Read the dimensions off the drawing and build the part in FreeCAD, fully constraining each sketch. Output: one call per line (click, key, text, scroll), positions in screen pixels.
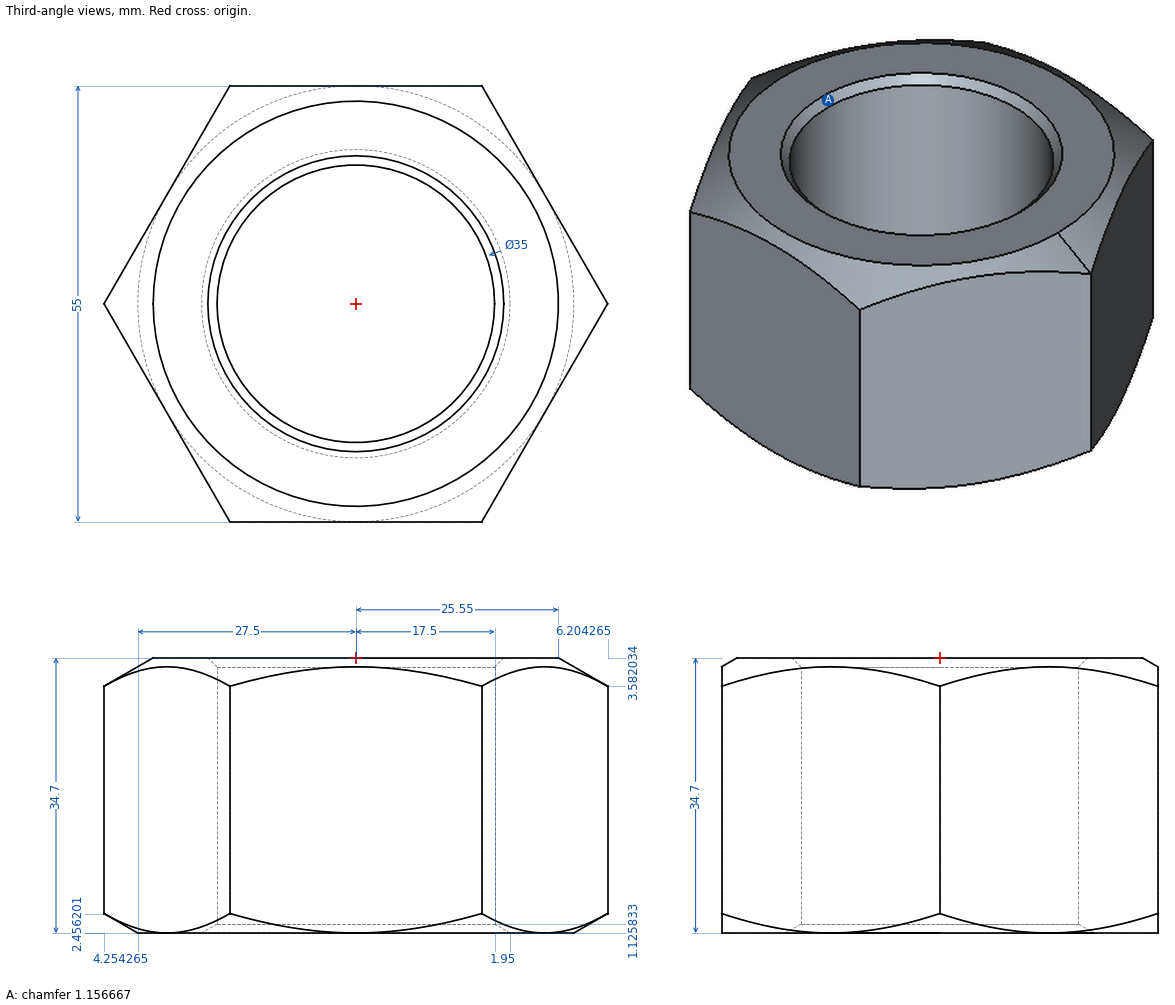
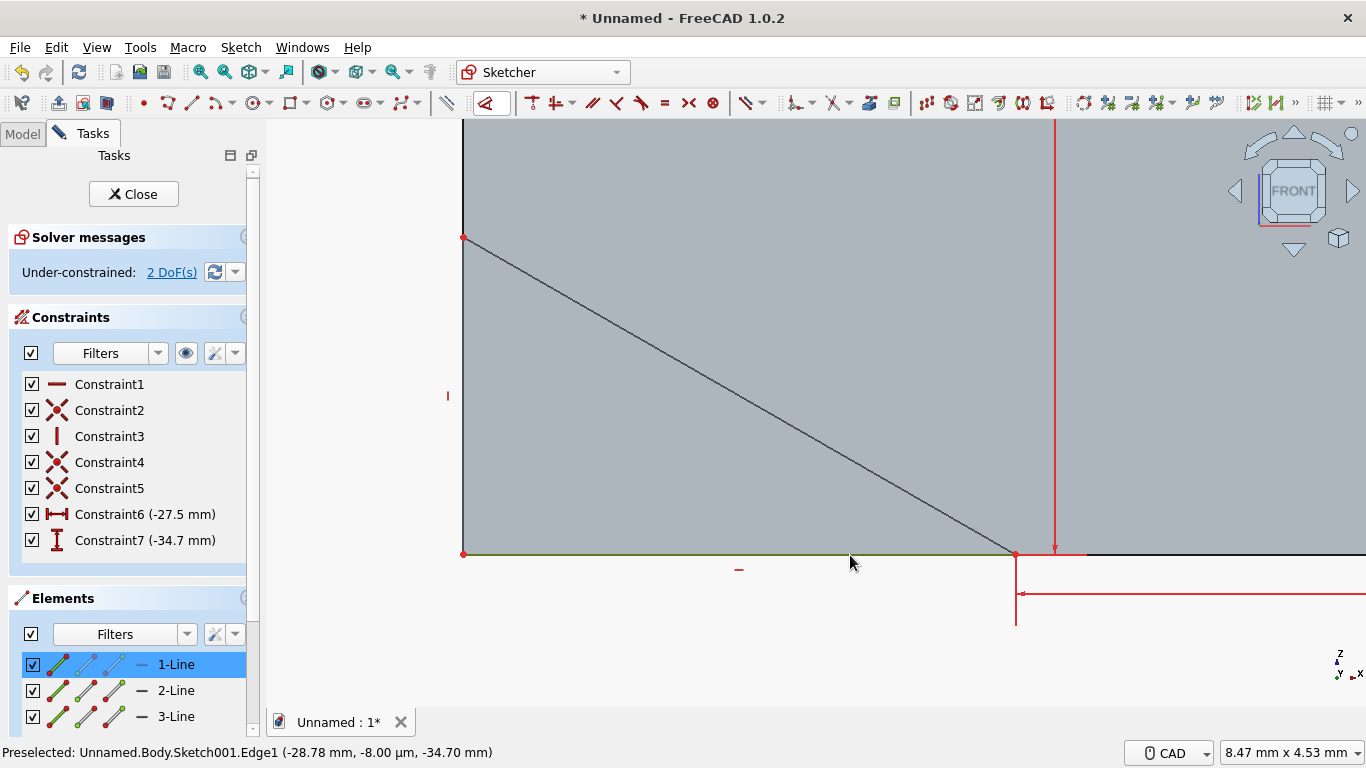
key(l)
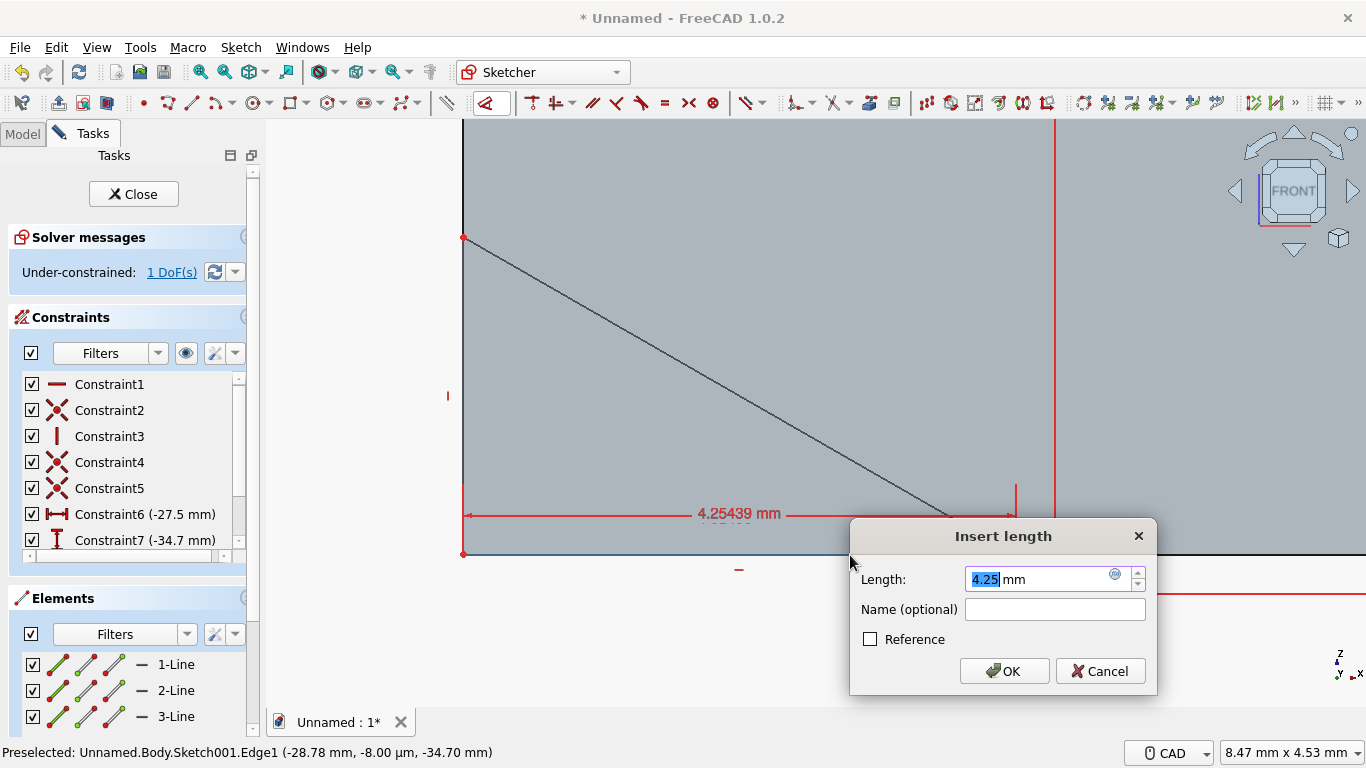
text(4.254265)
key(Return)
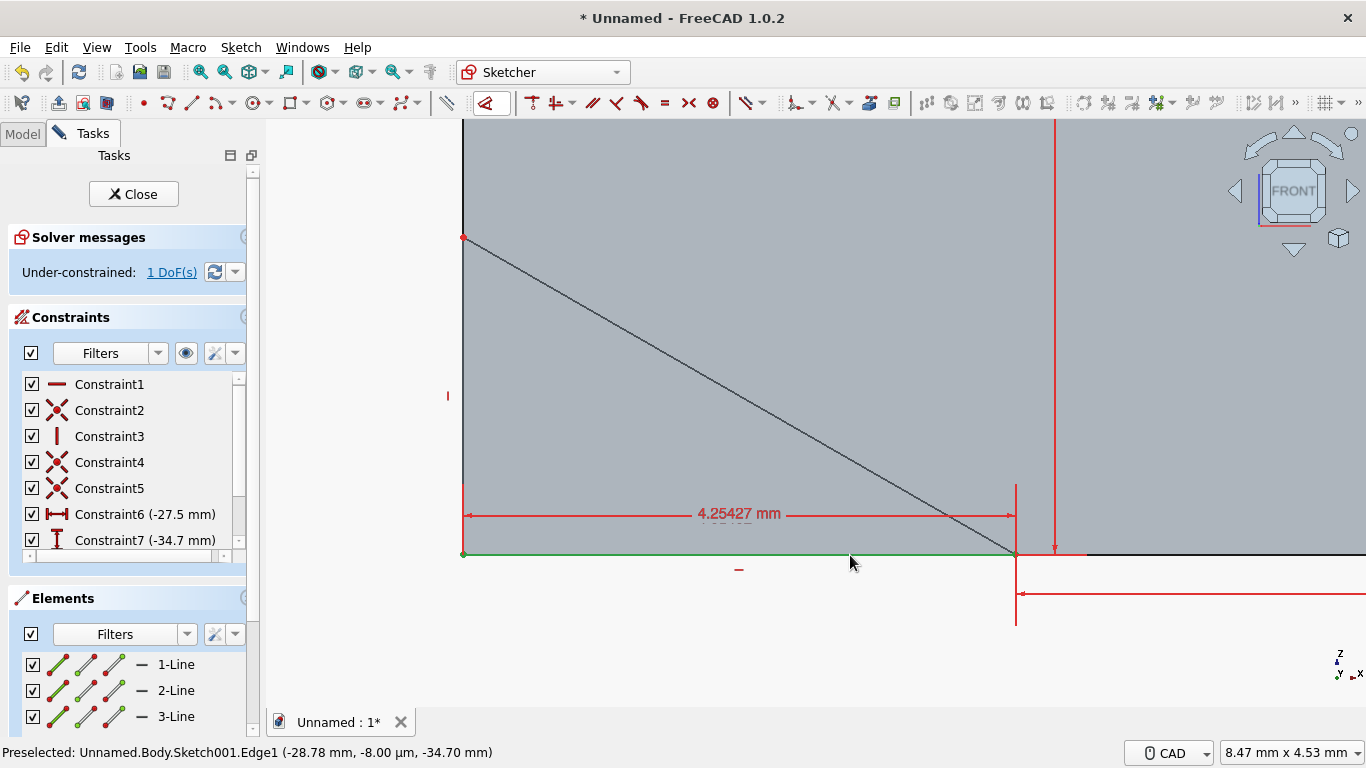
click(463, 459)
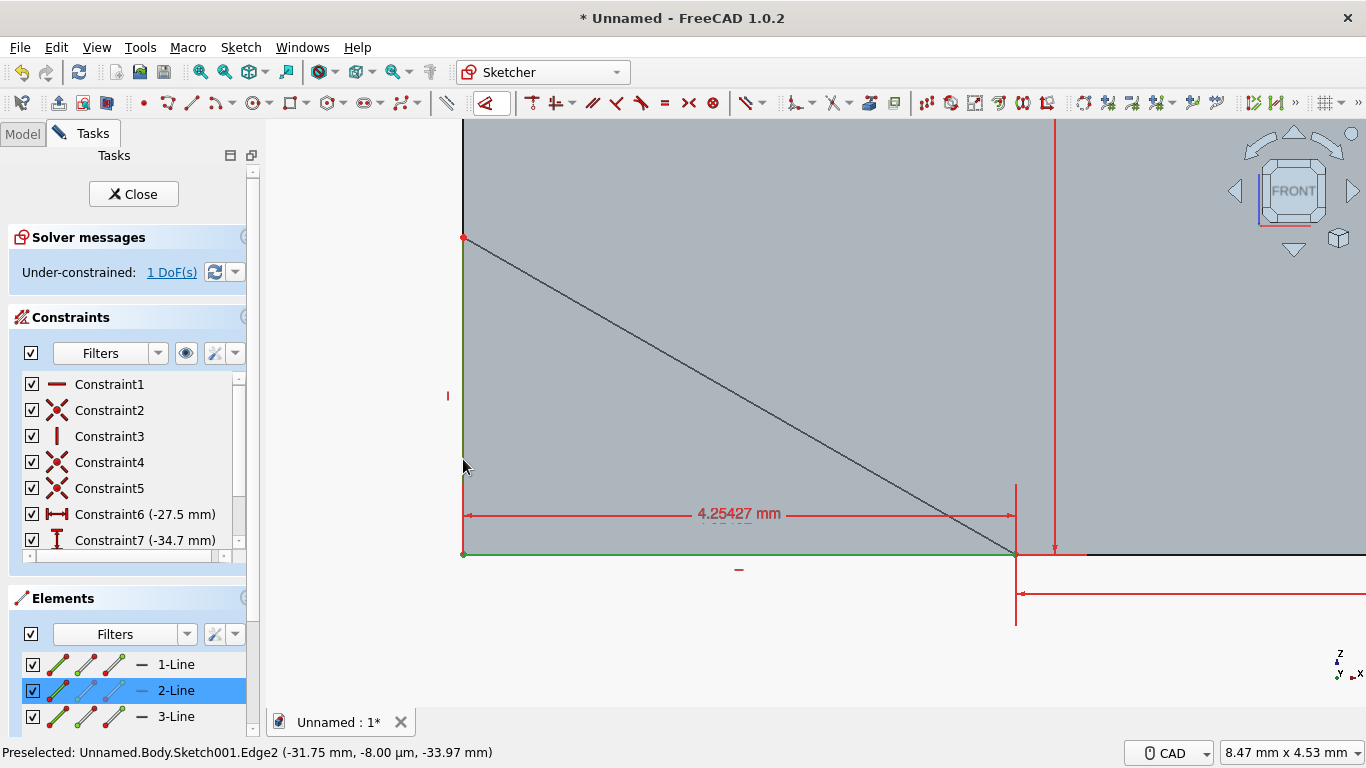
key(i)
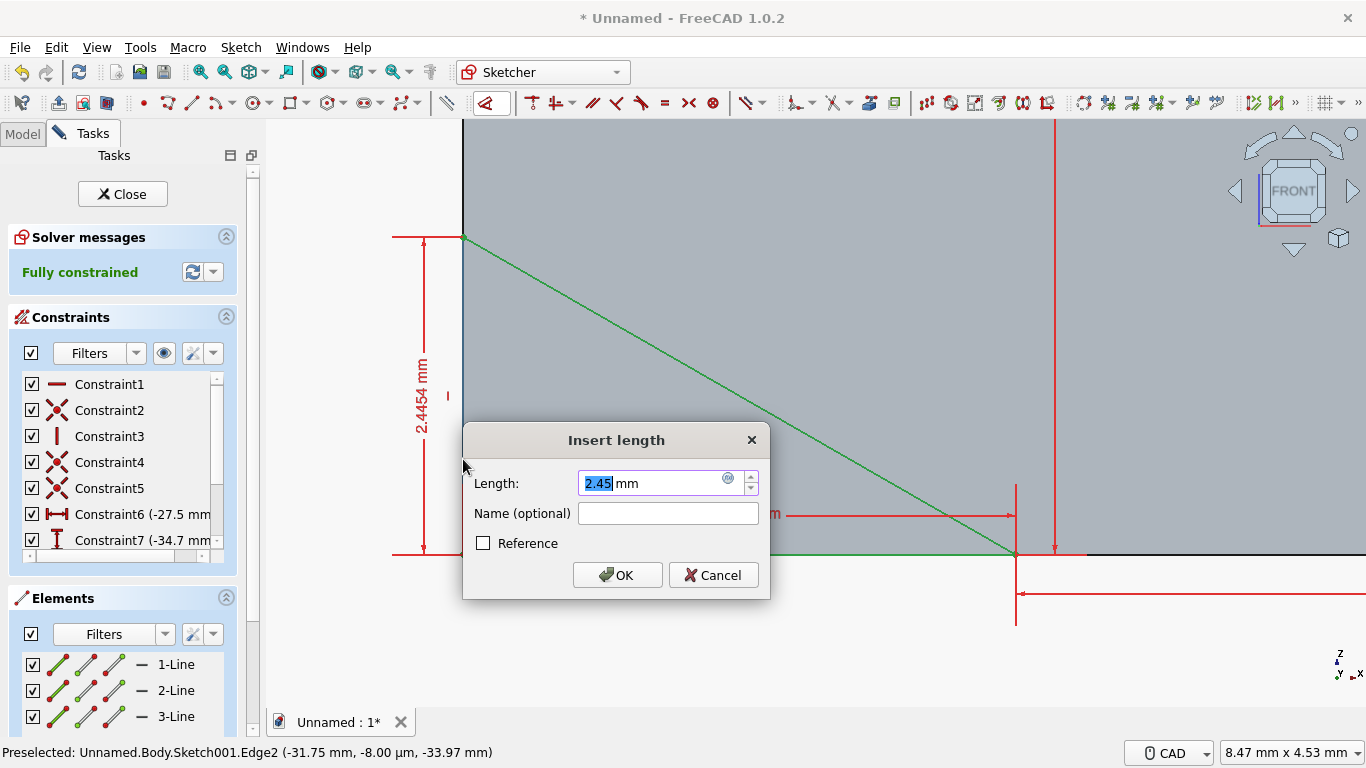
text(2.456201)
key(Return)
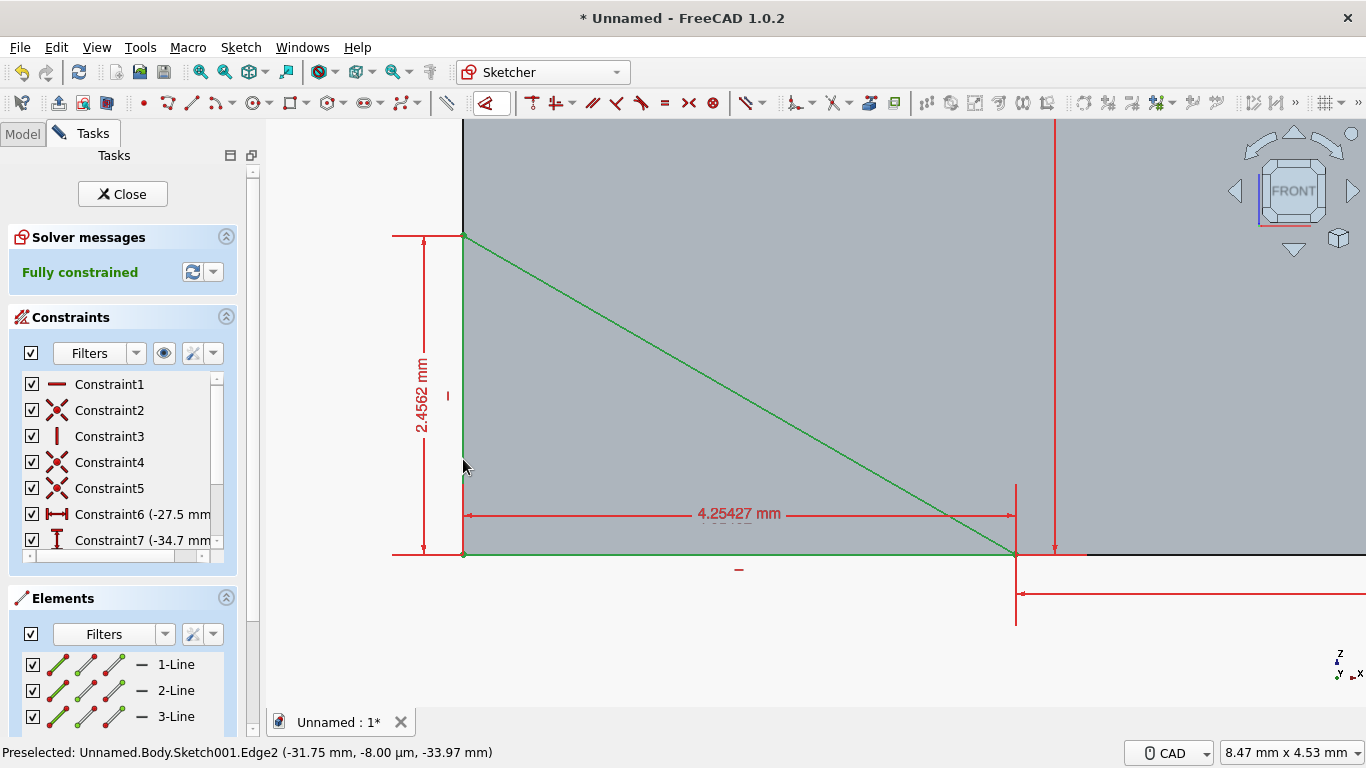
click(123, 194)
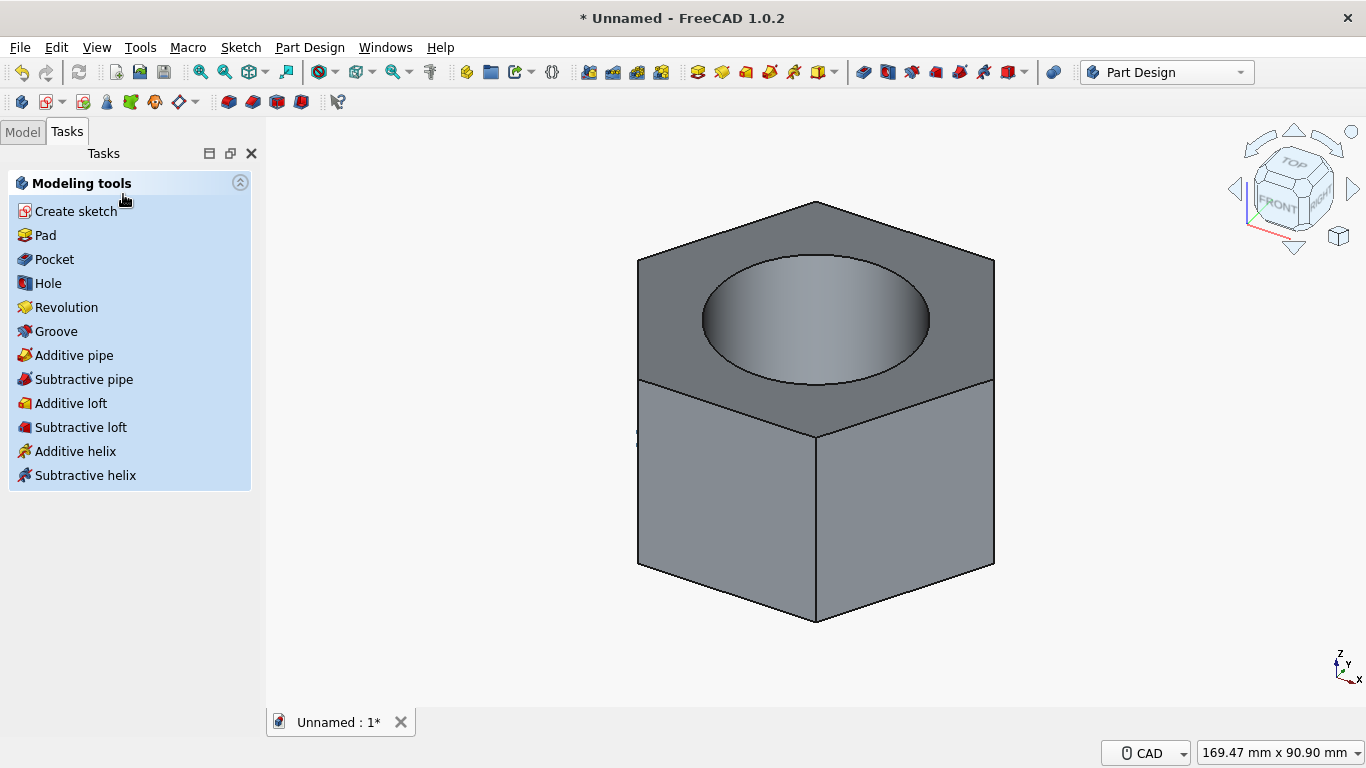
click(912, 72)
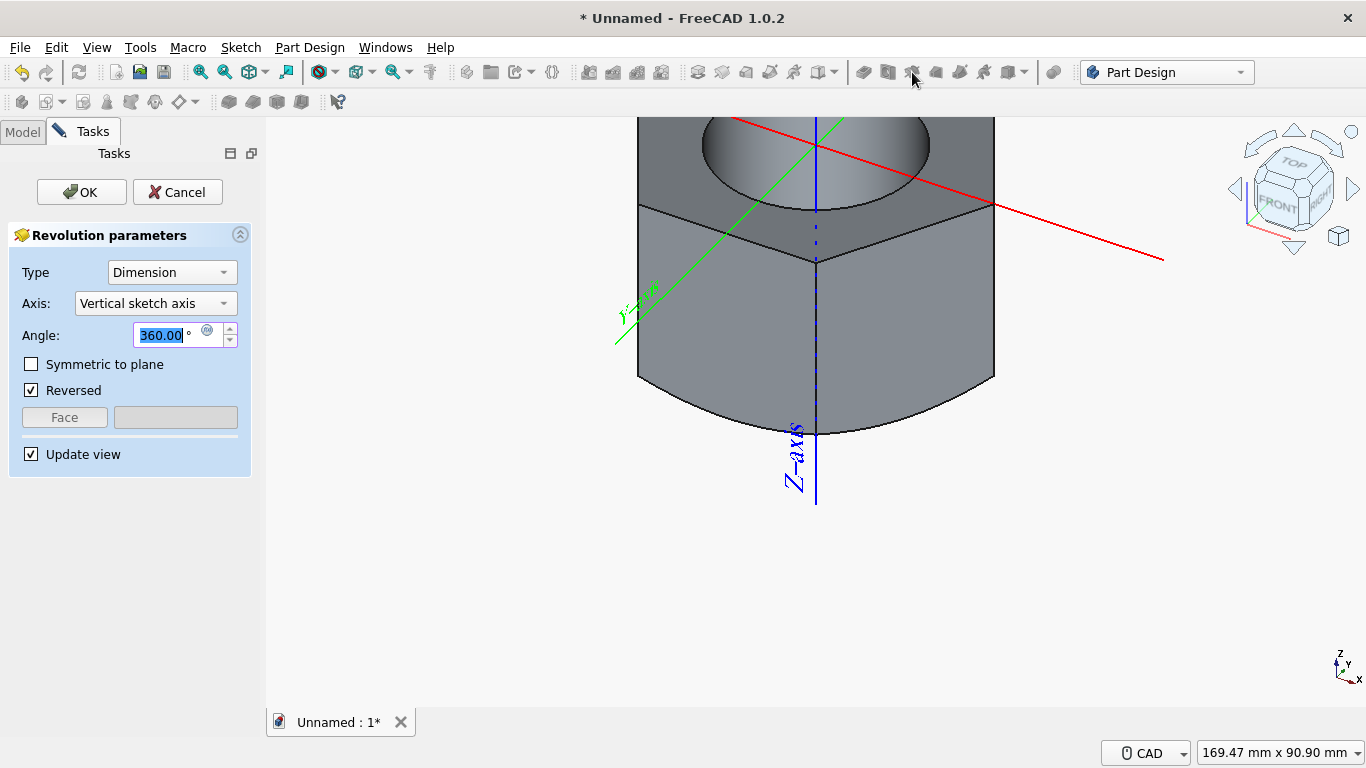
click(82, 192)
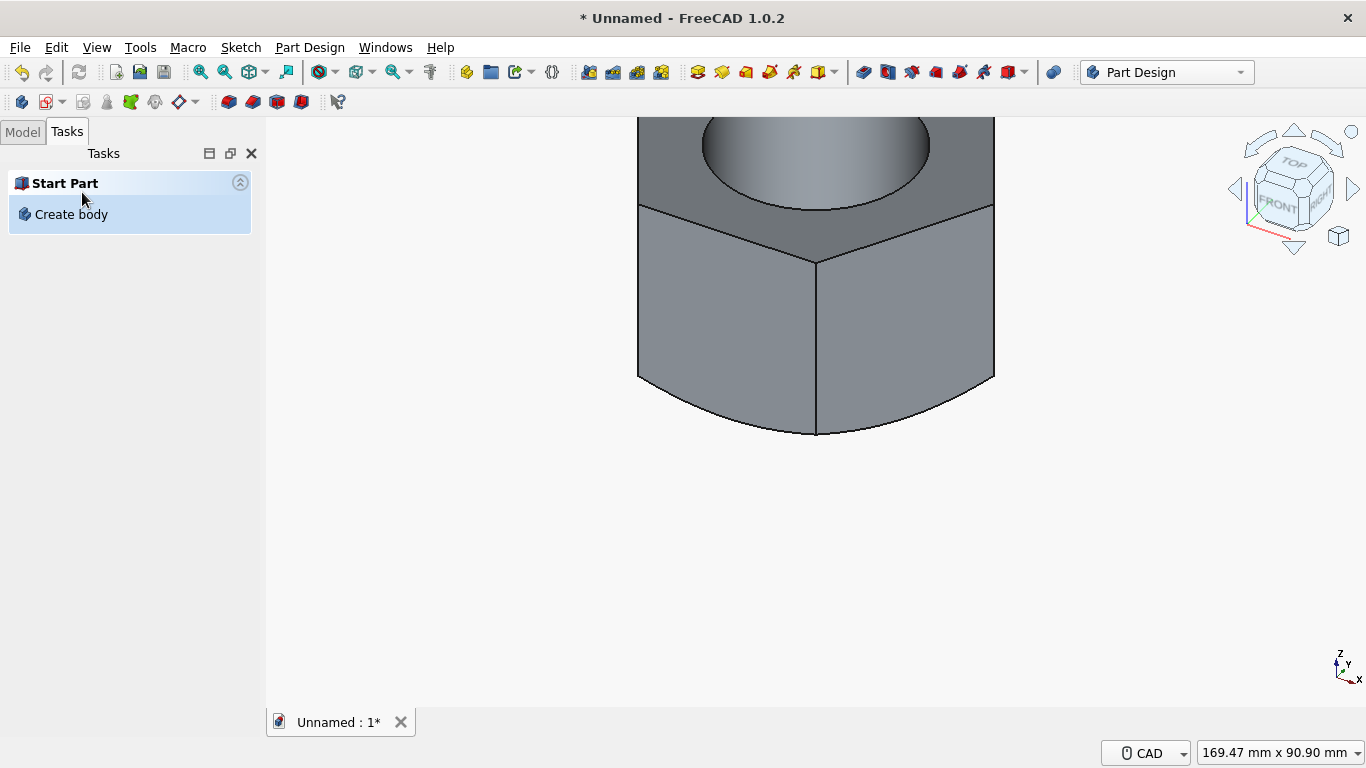
key(v)
key(f)